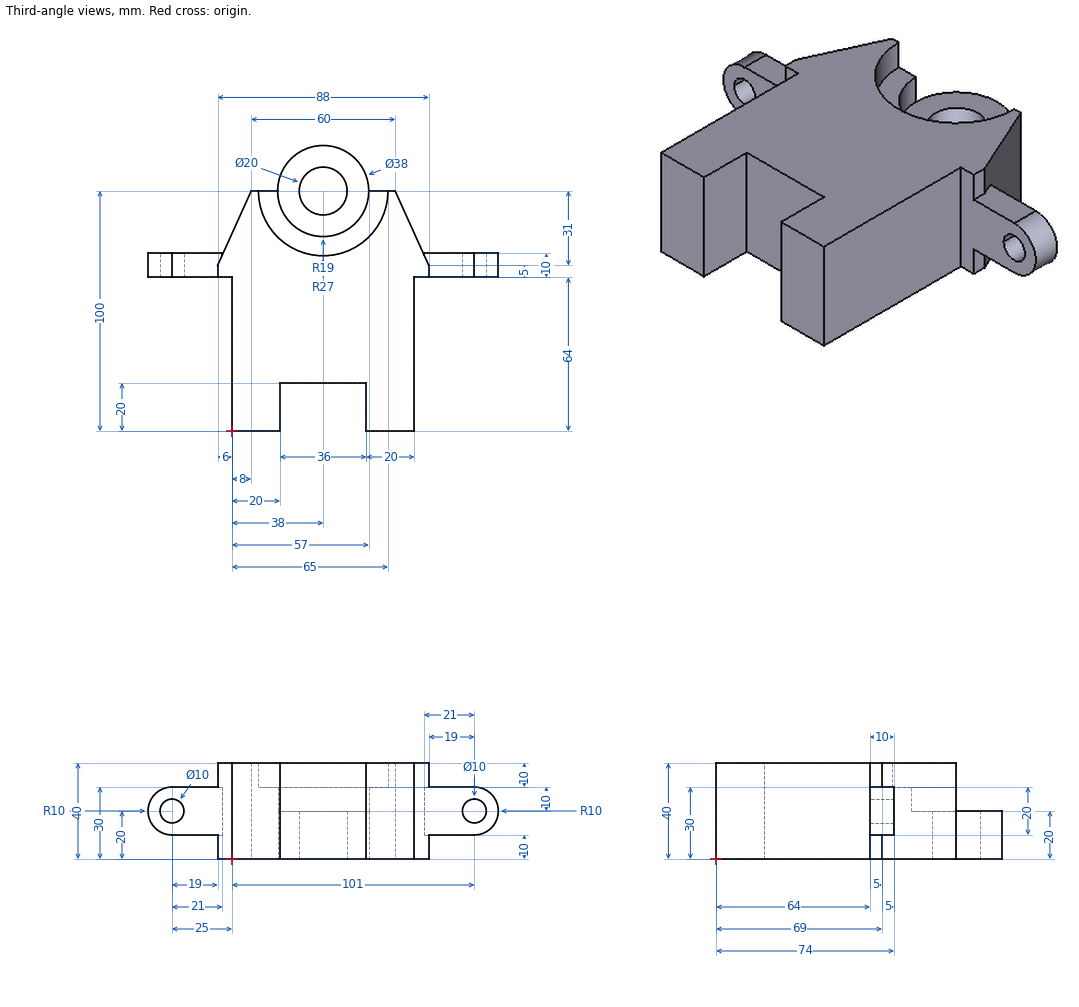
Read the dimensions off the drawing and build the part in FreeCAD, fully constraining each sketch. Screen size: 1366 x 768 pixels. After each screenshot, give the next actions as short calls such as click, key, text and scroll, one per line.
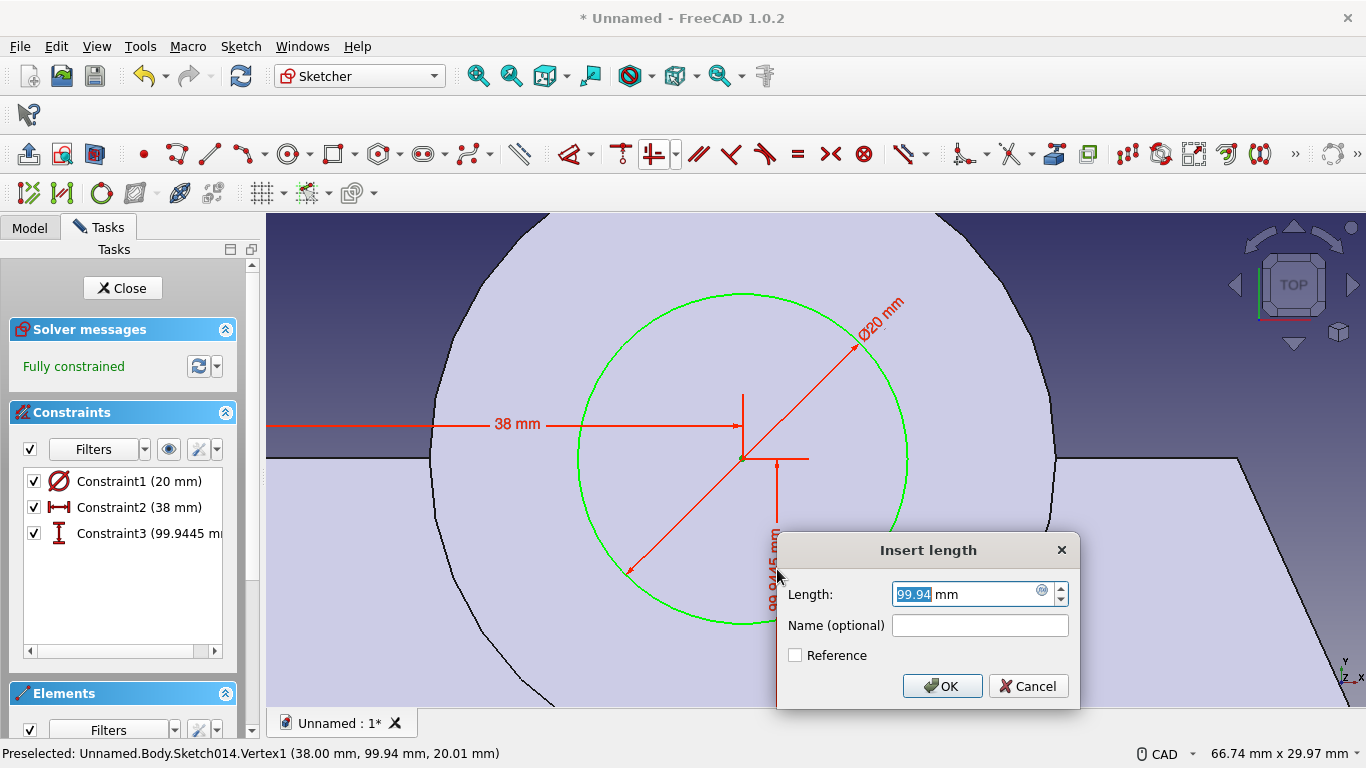
text(100)
key(Return)
key(Escape)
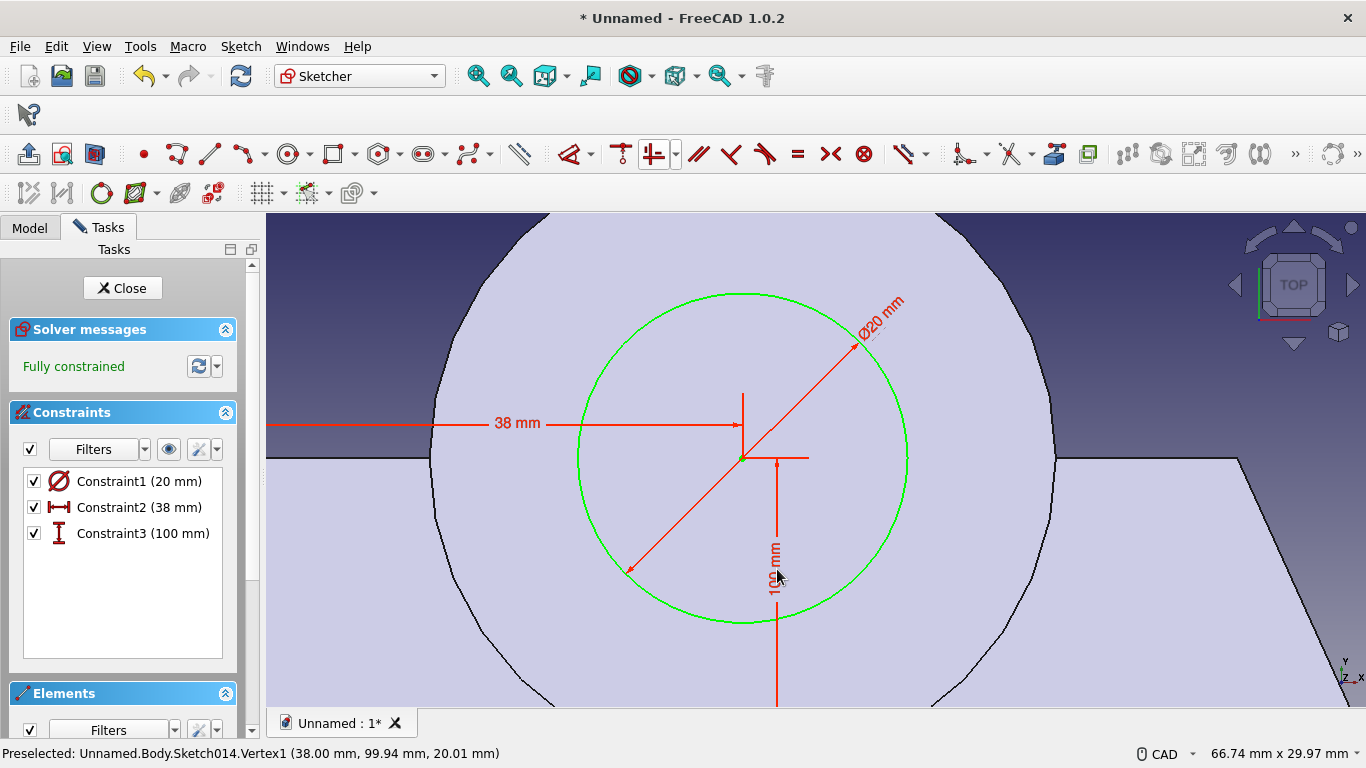
click(123, 288)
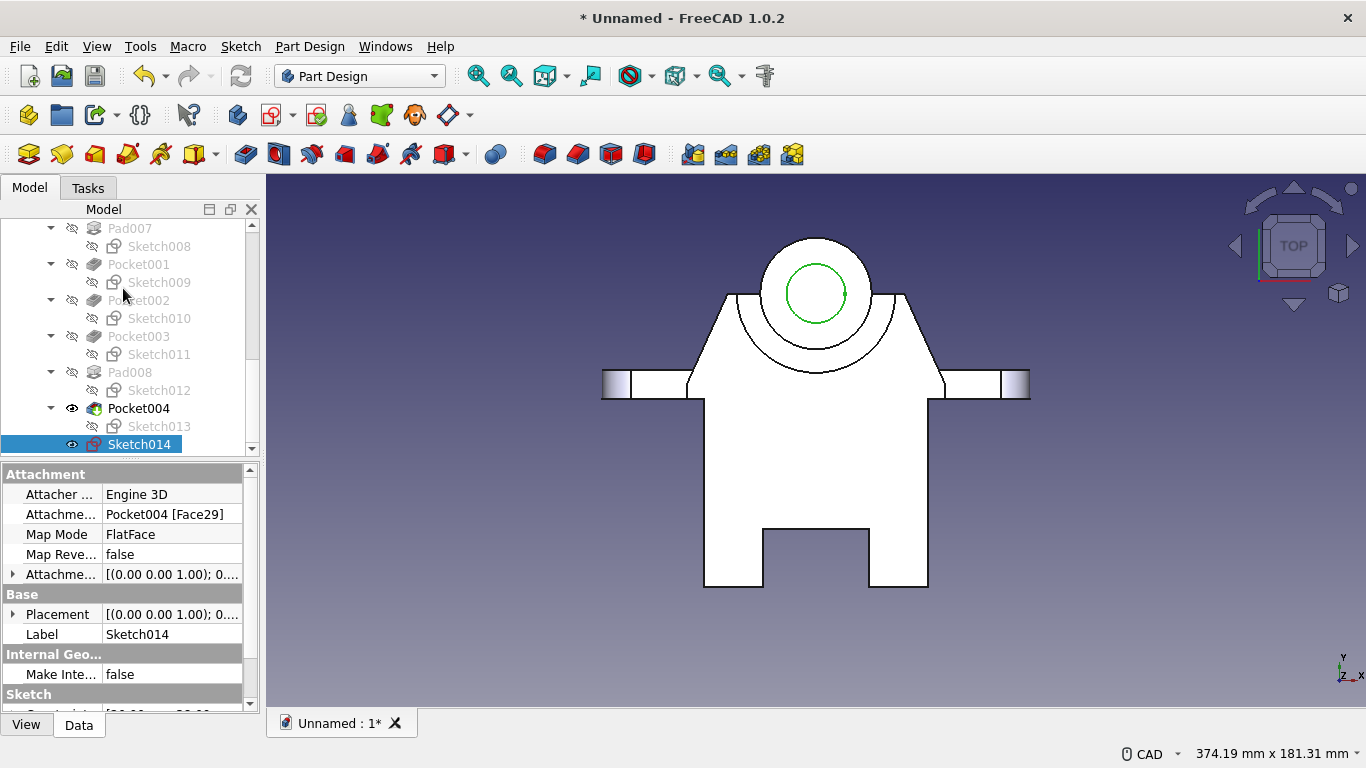
click(246, 154)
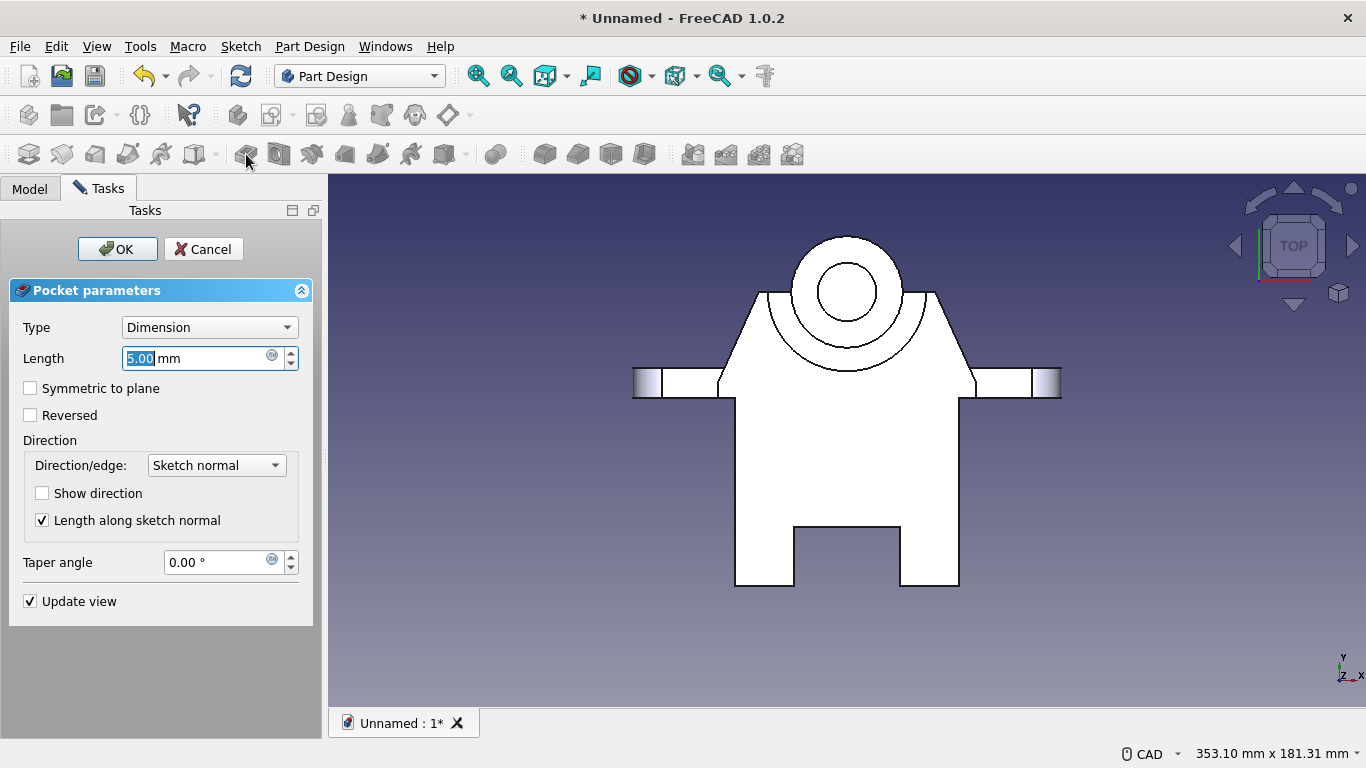
text(20)
key(Tab)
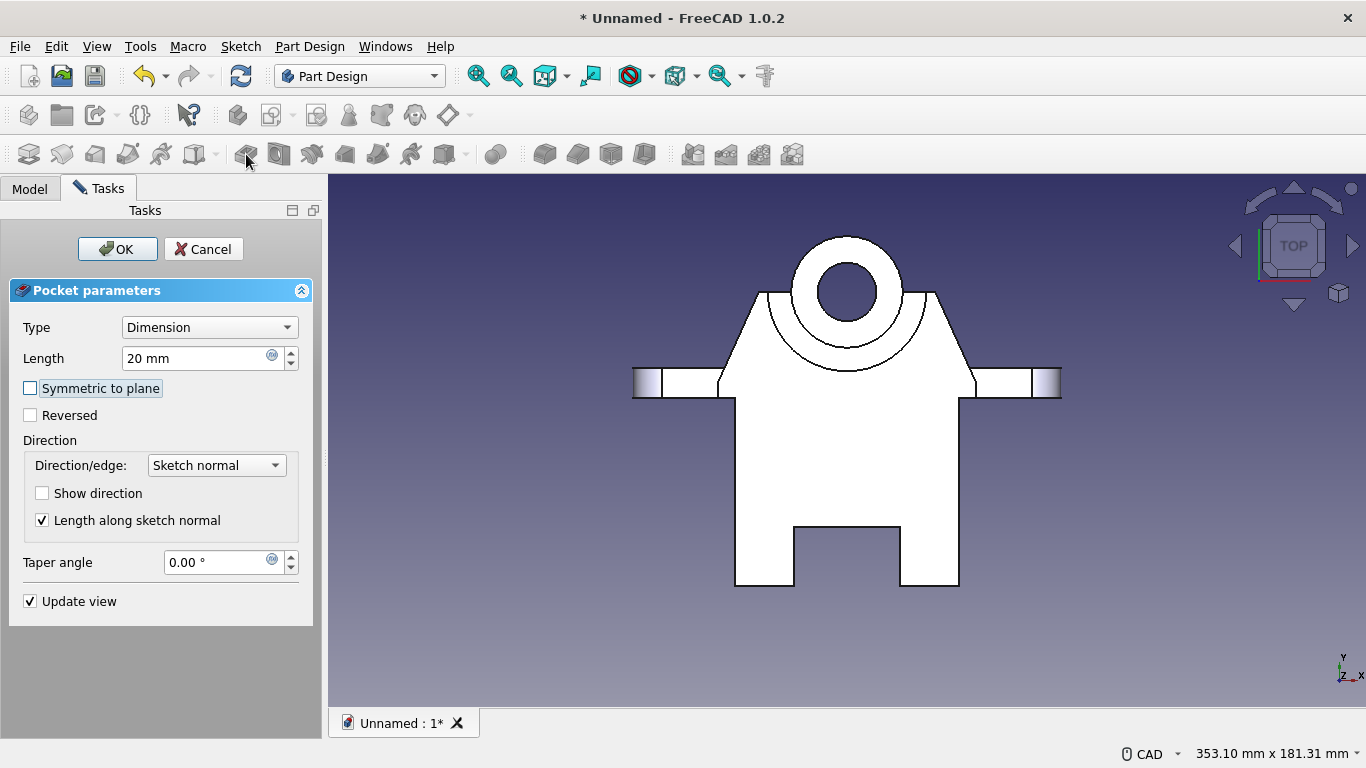
click(118, 249)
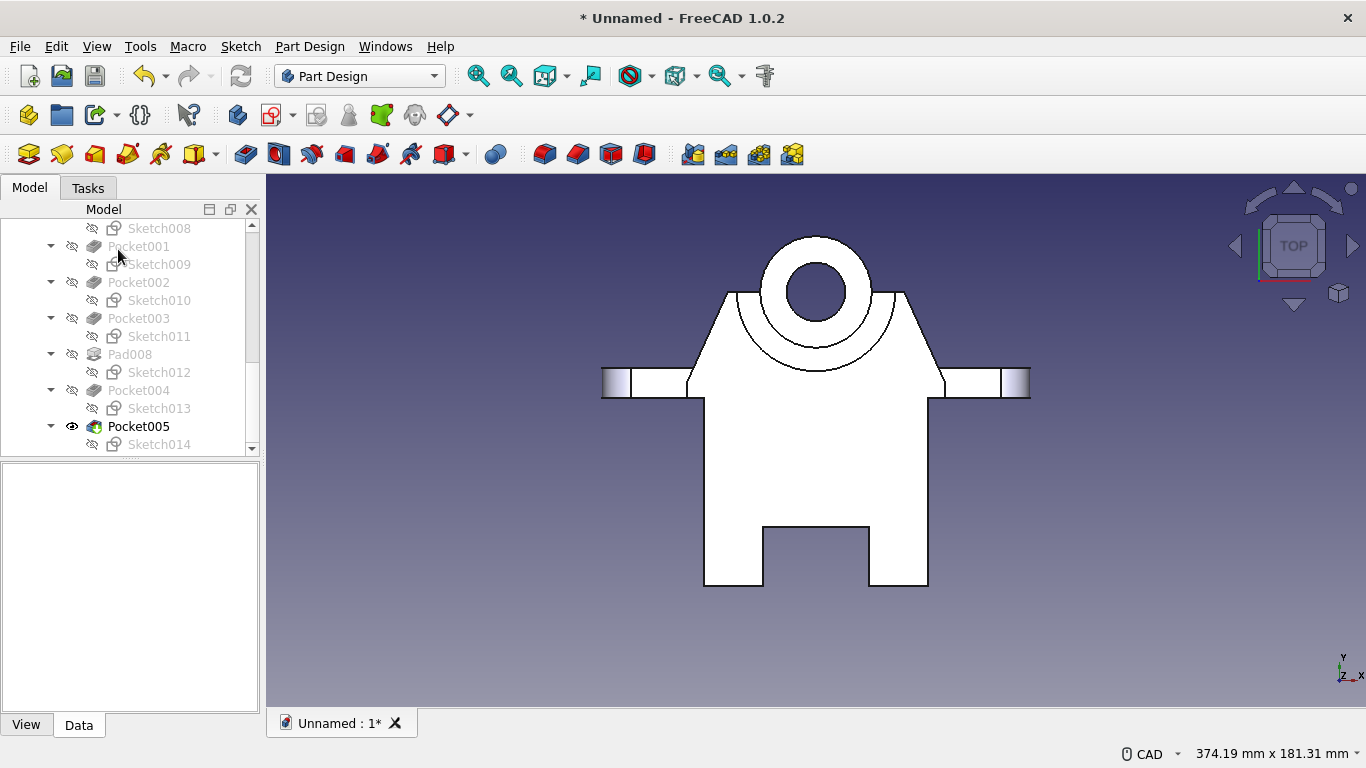
key(0)